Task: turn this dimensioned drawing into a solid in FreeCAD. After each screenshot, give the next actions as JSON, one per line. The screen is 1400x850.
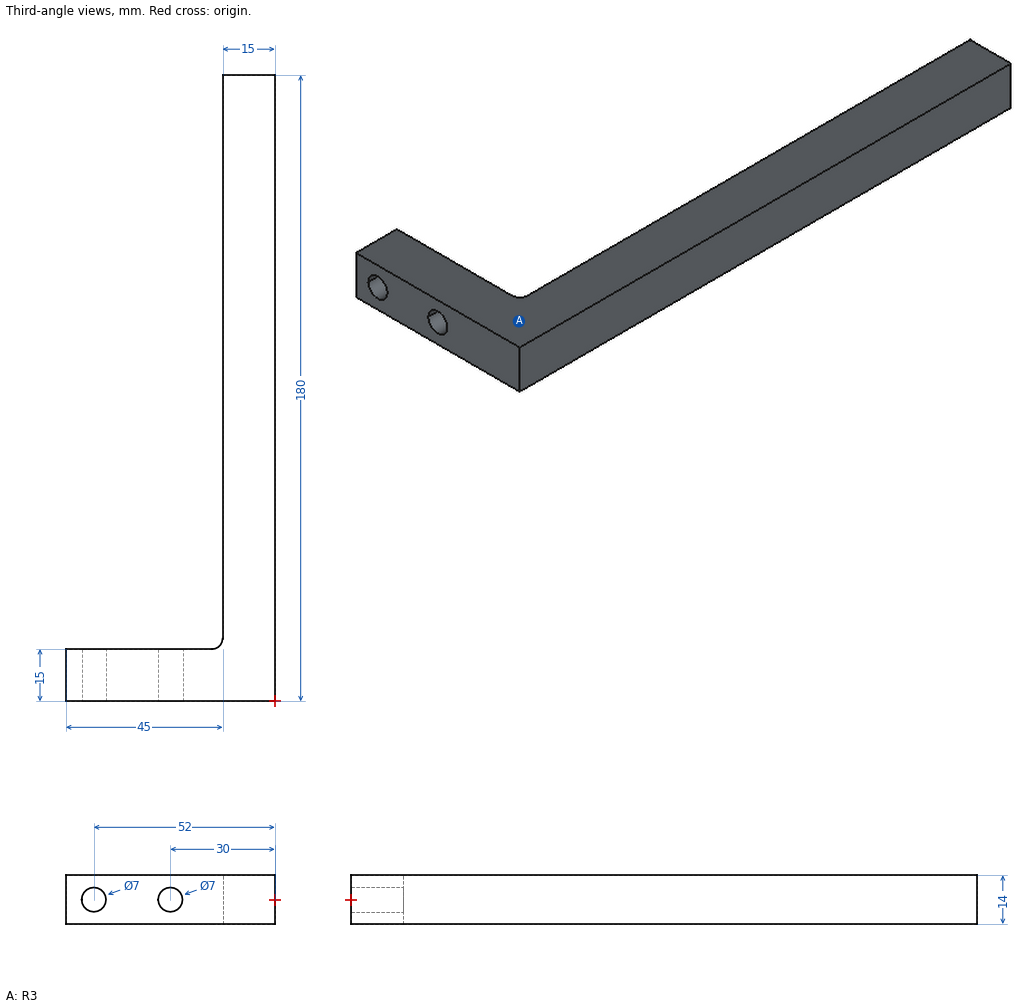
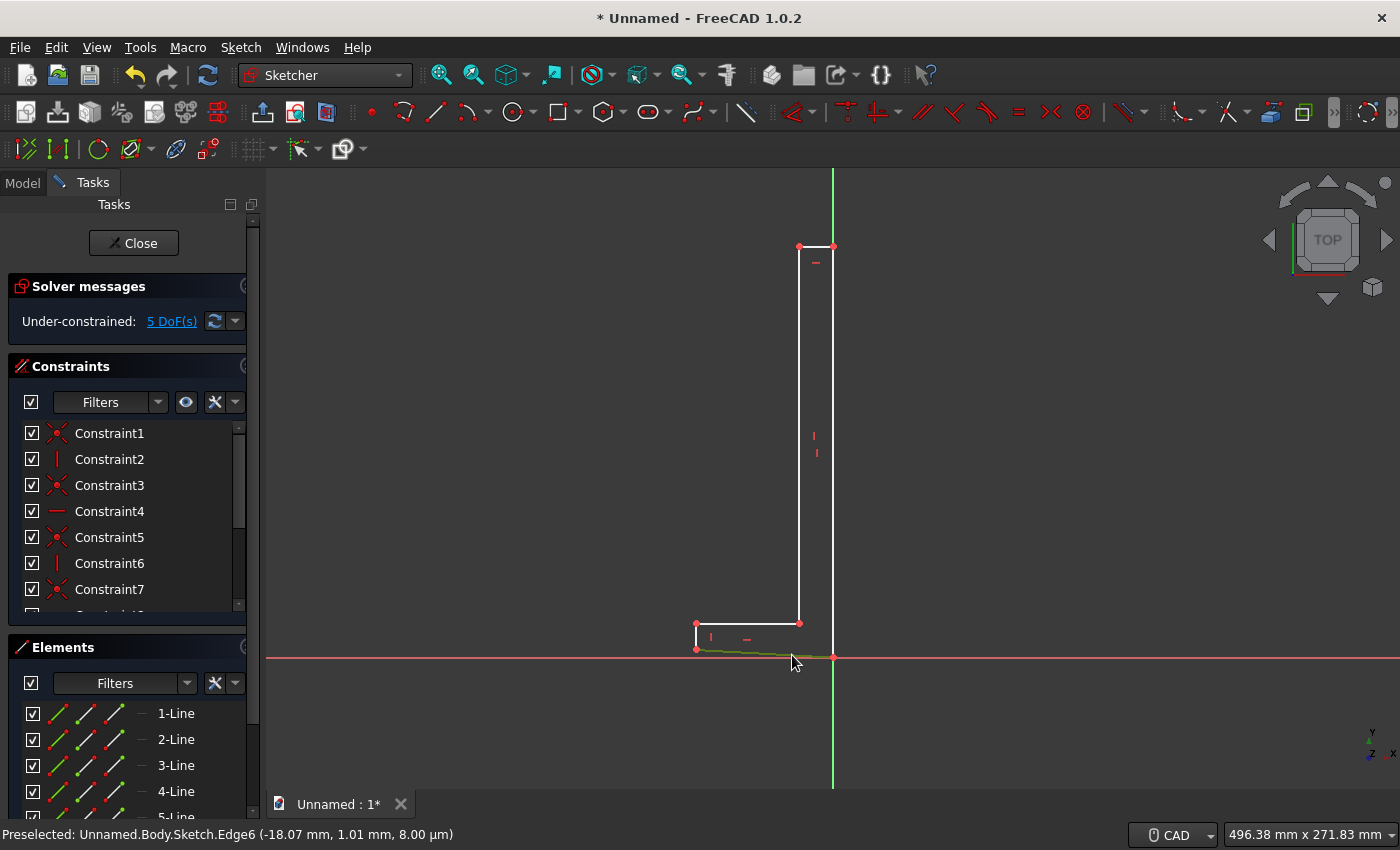
{"action": "left_click", "coordinate": [900, 112]}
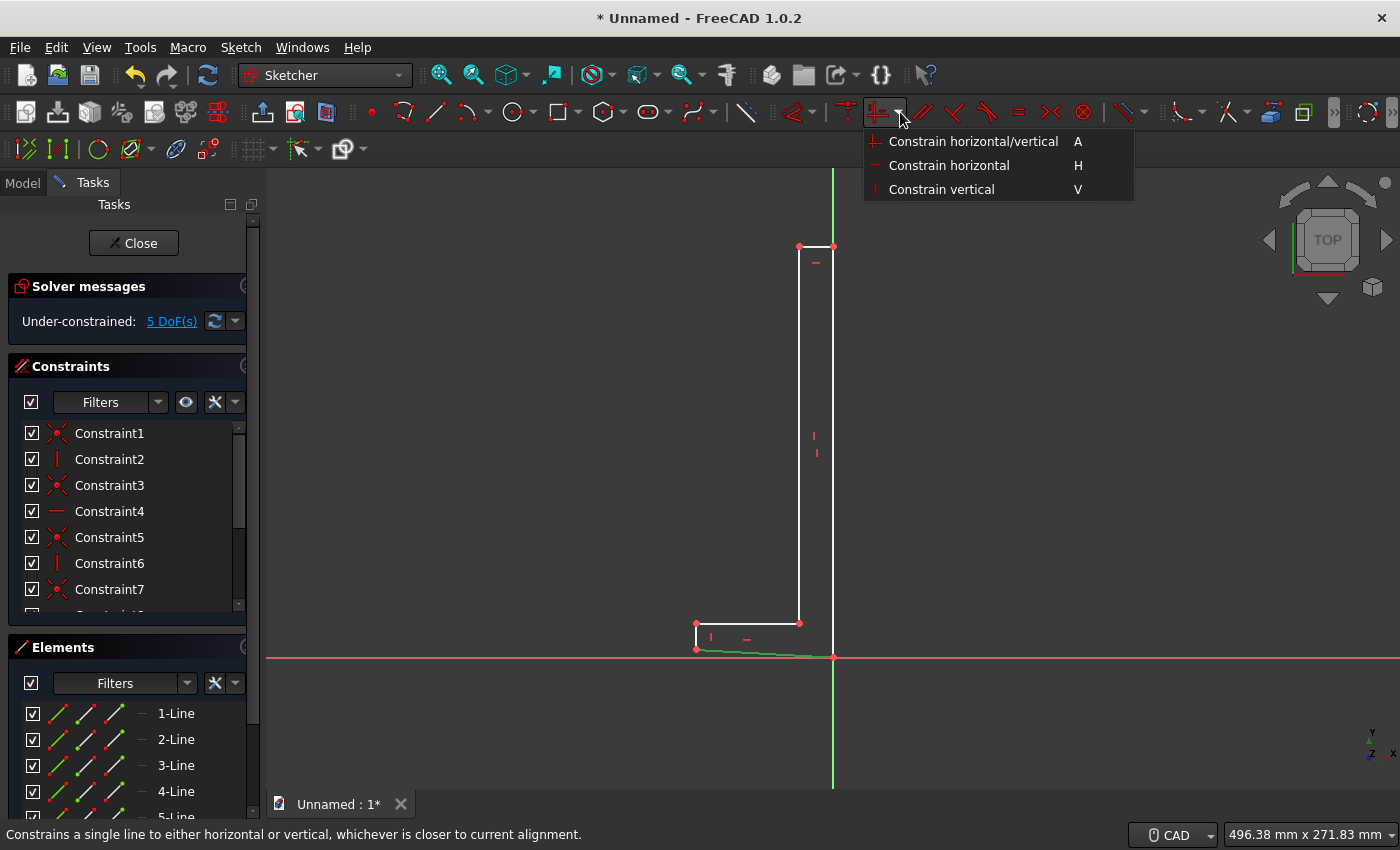
{"action": "left_click", "coordinate": [999, 165]}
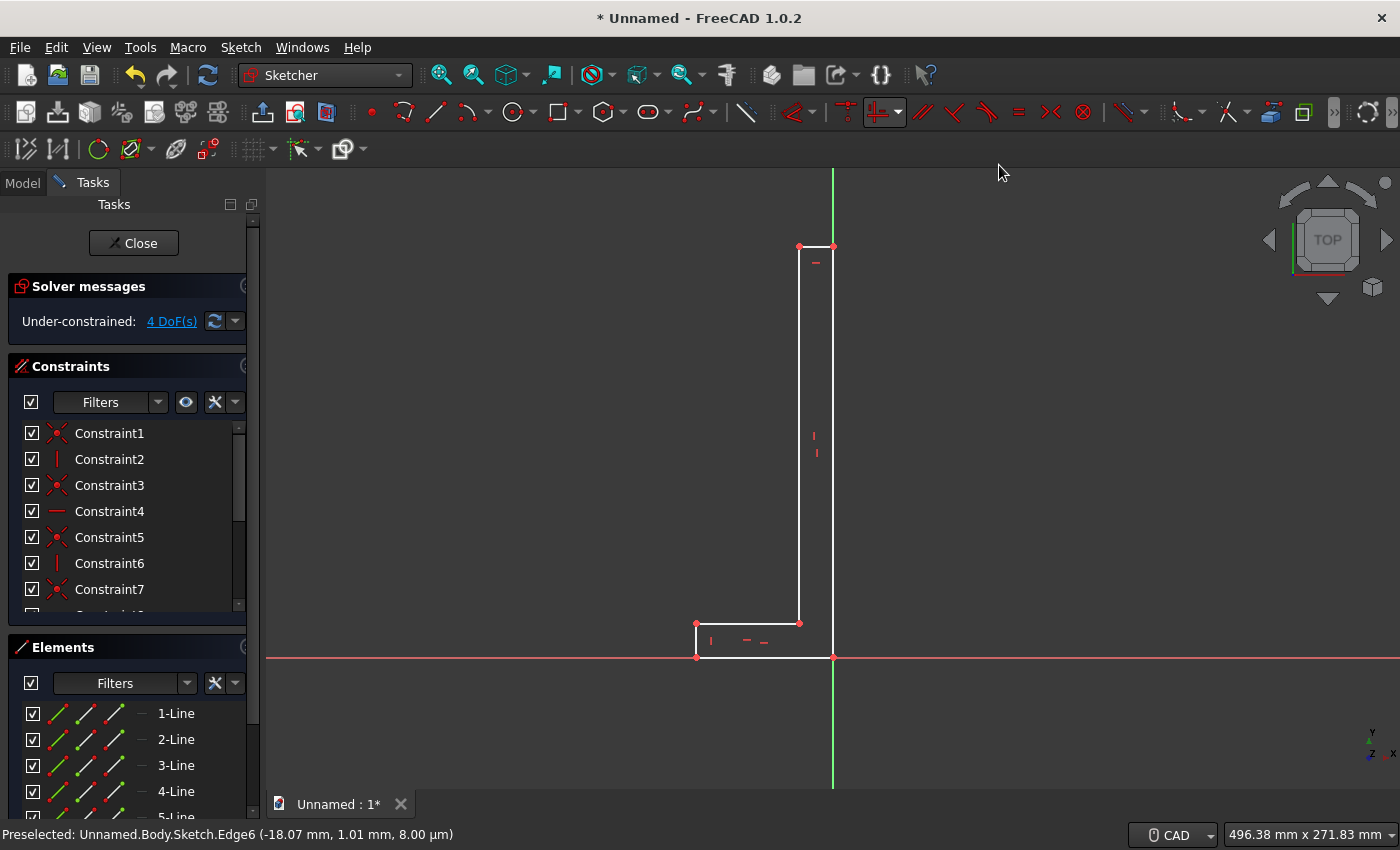
{"action": "scroll", "coordinate": [823, 247], "scroll_direction": "up", "scroll_amount": 2}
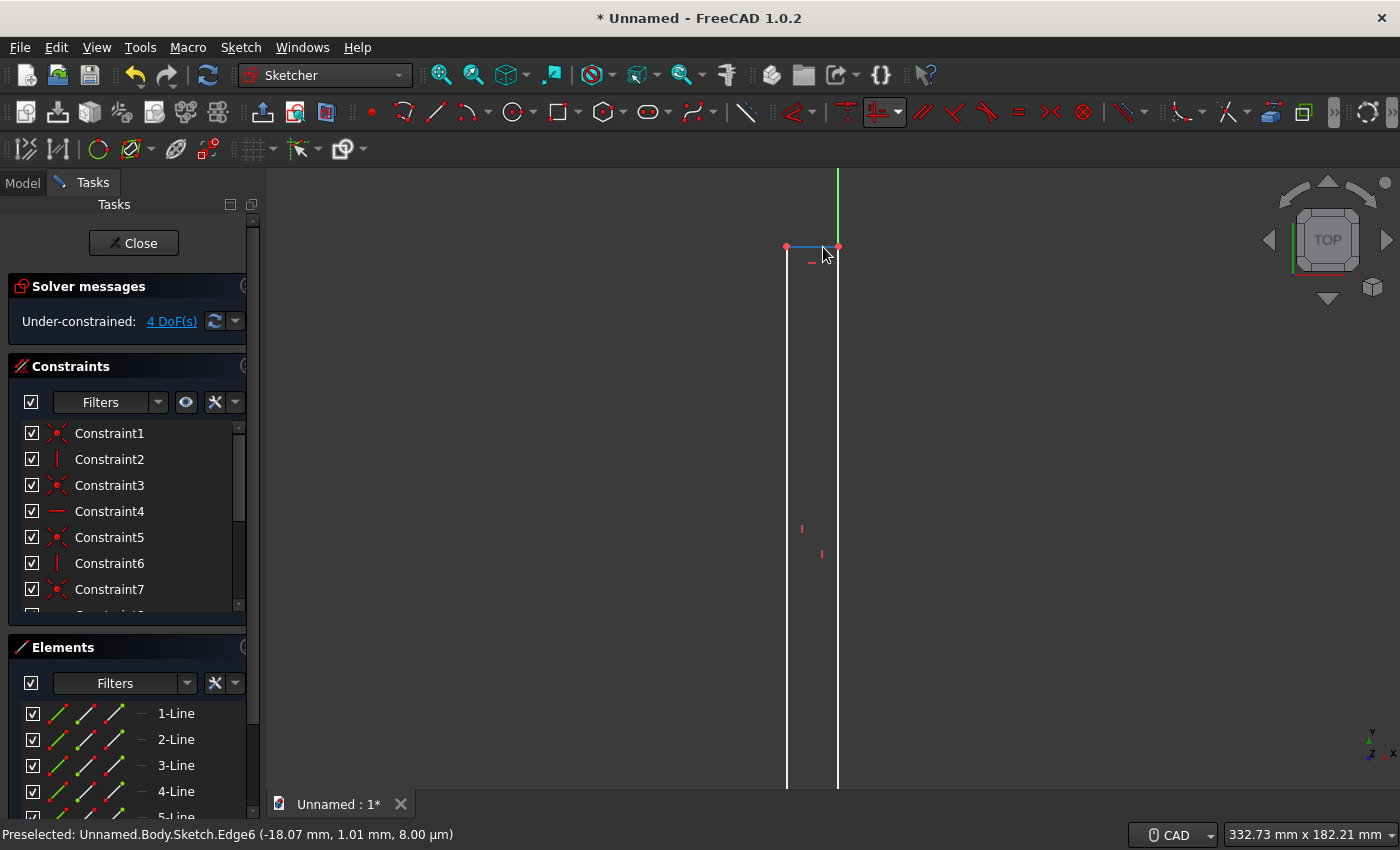
{"action": "left_click", "coordinate": [823, 247]}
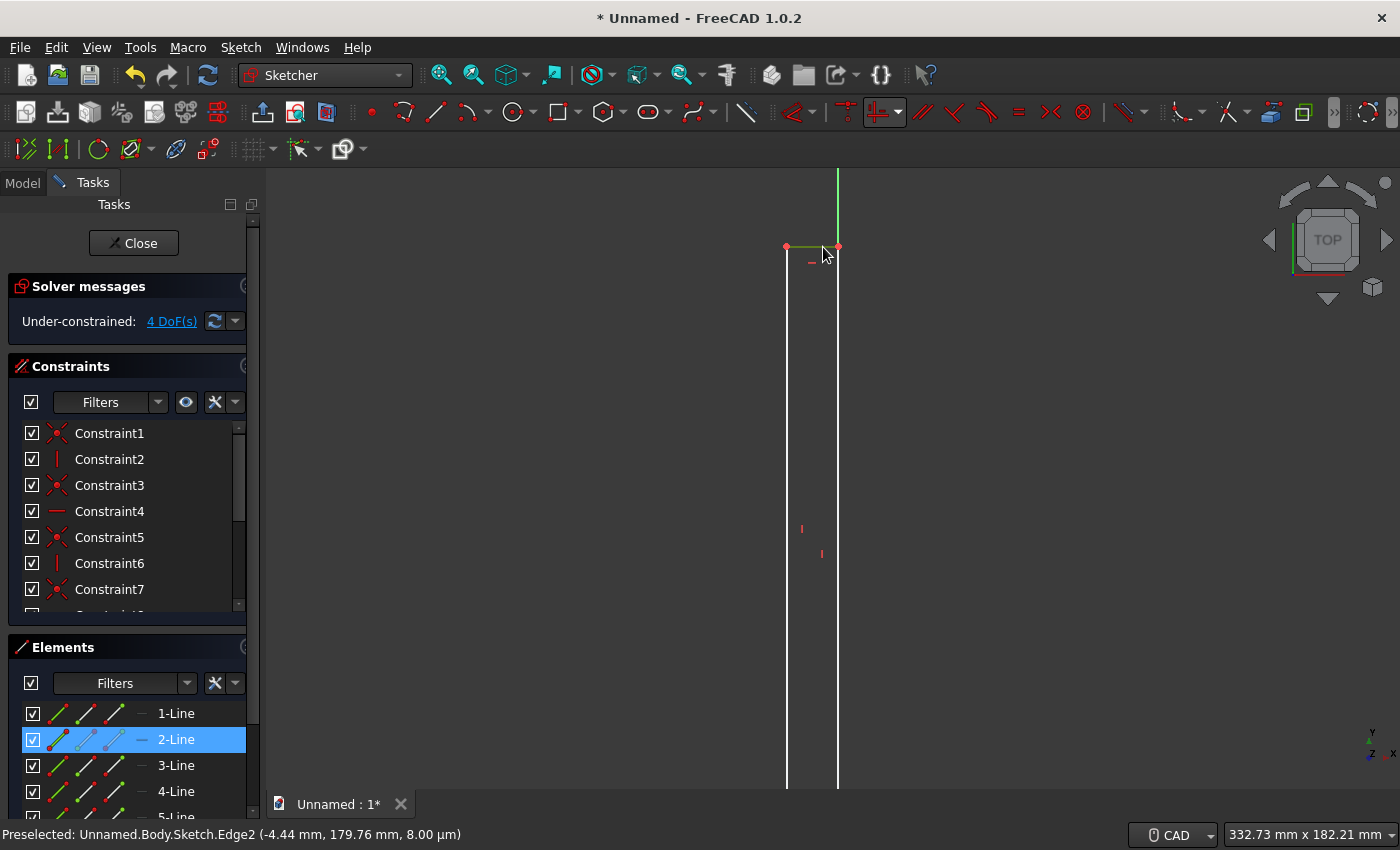
{"action": "key", "text": "l"}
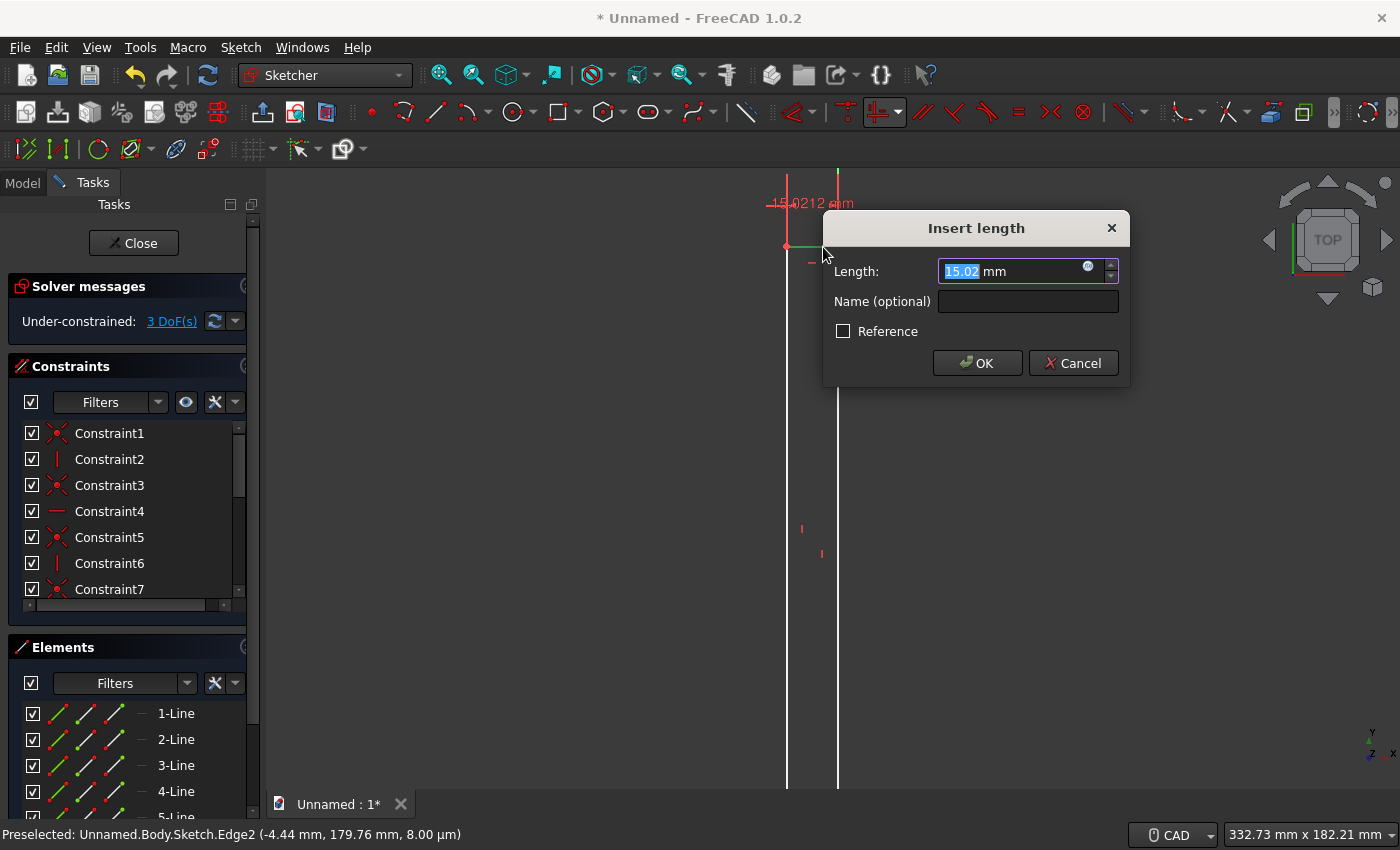
{"action": "type", "text": "15"}
{"action": "key", "text": "Return"}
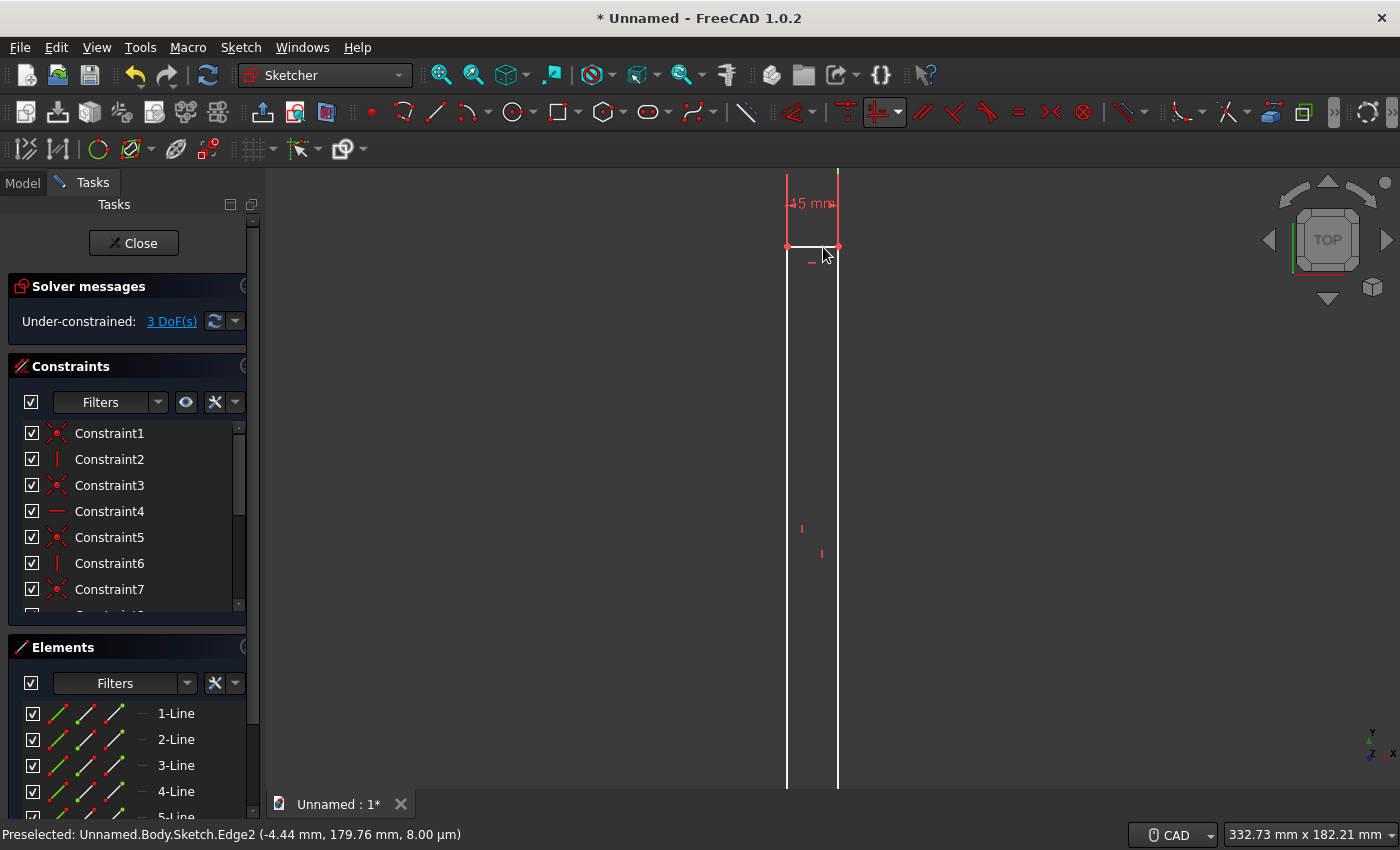
{"action": "scroll", "coordinate": [823, 327], "scroll_direction": "down", "scroll_amount": 2}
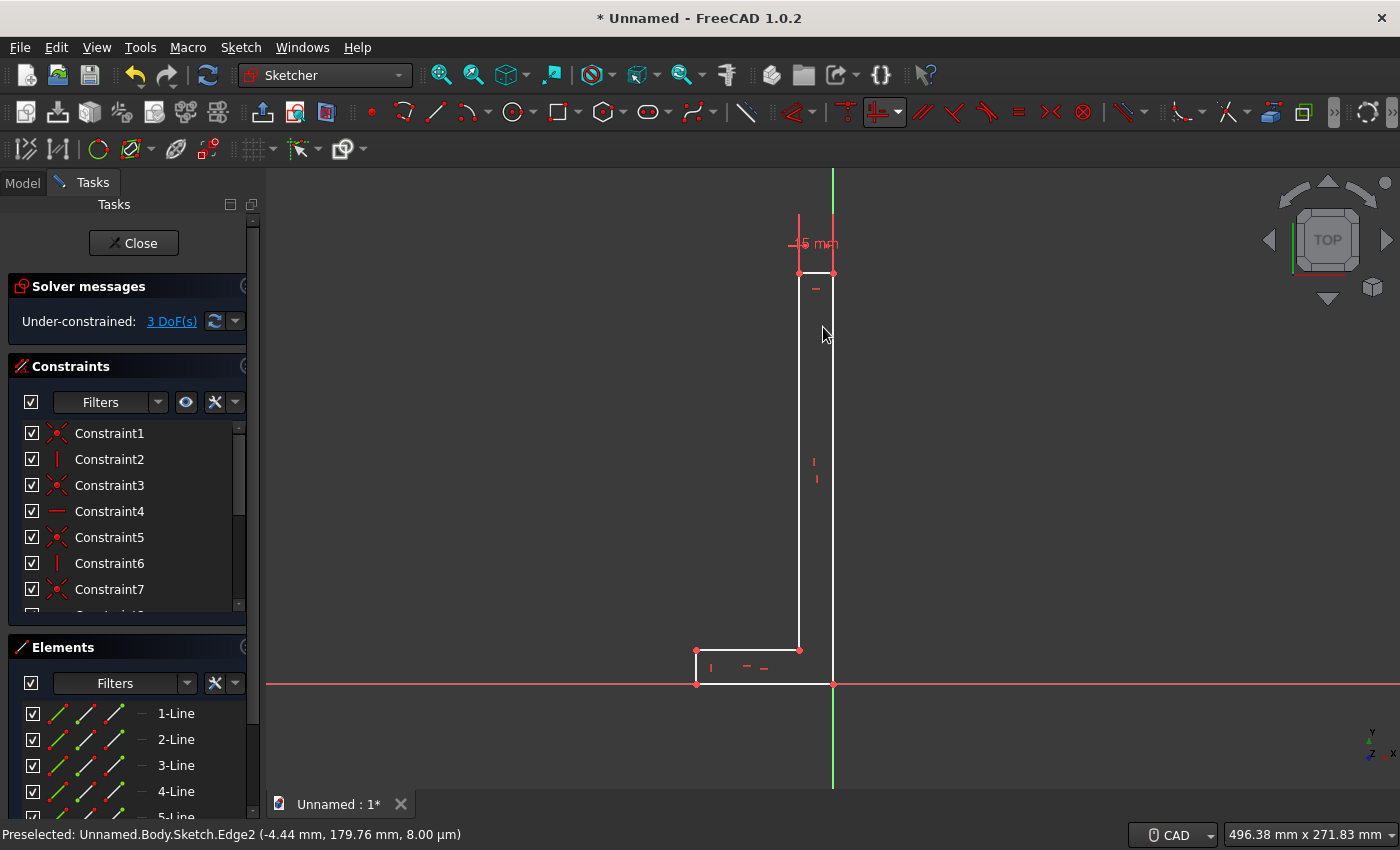
{"action": "left_click", "coordinate": [768, 650]}